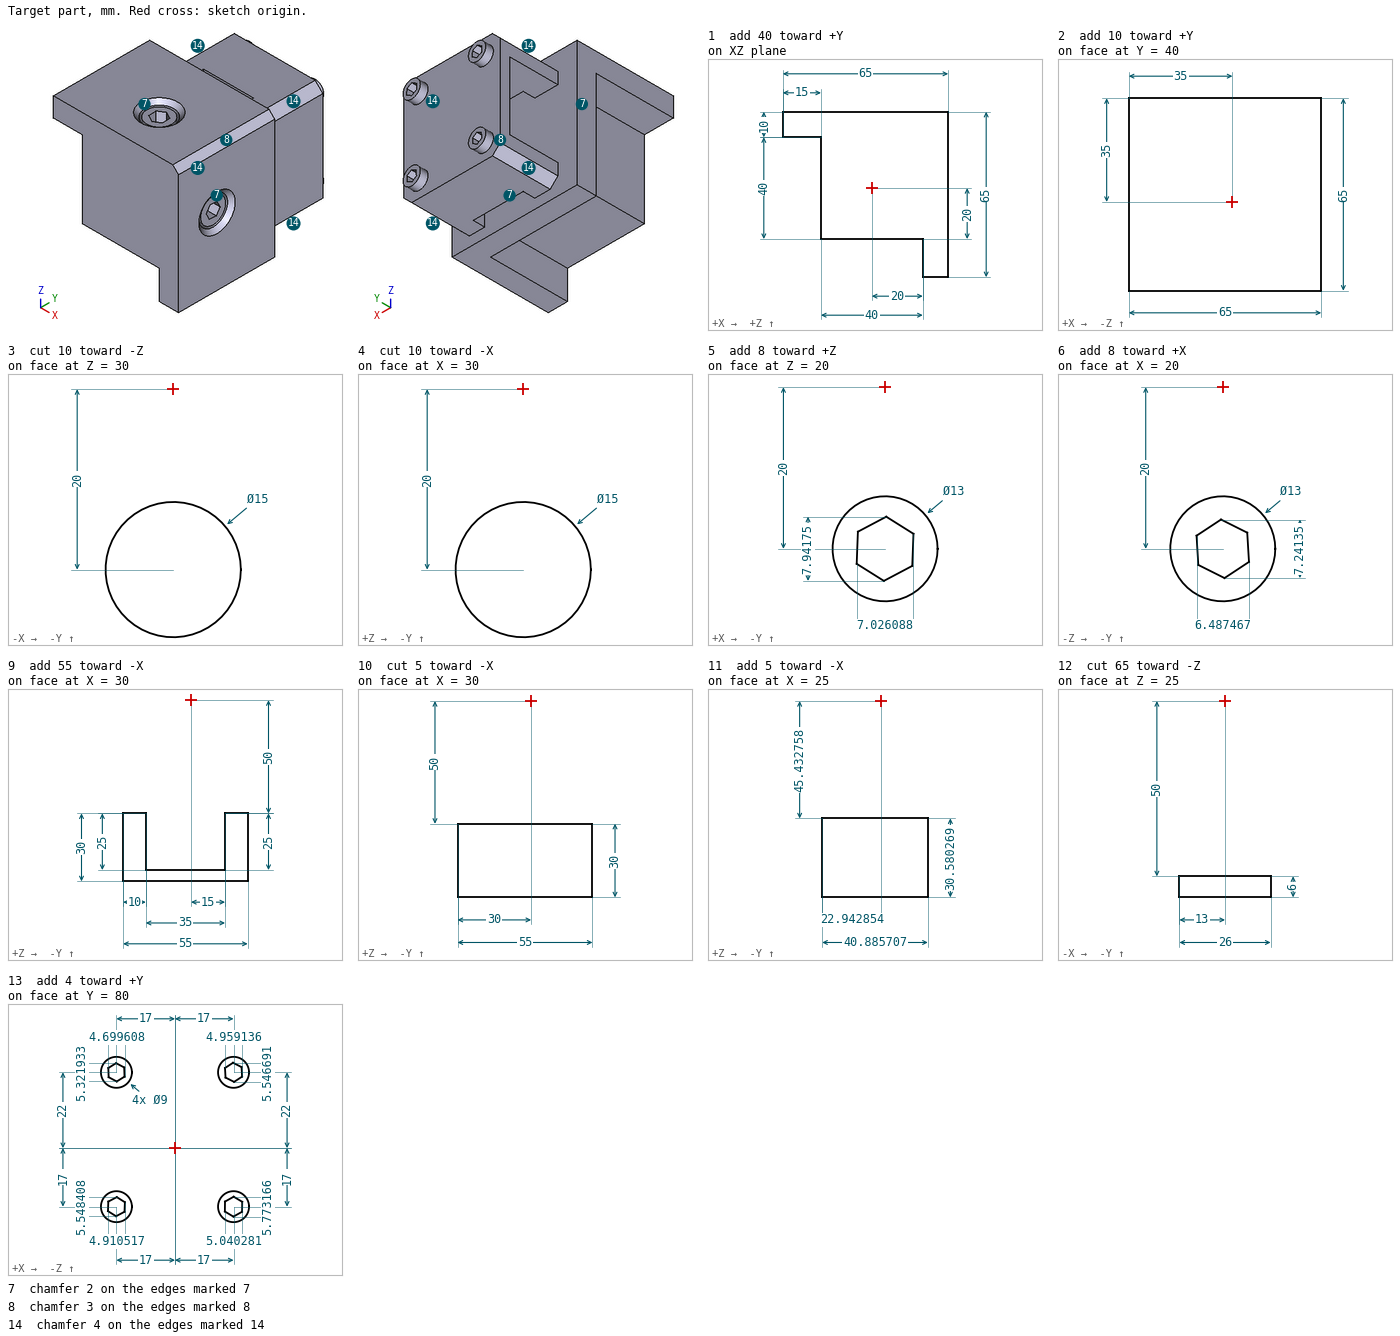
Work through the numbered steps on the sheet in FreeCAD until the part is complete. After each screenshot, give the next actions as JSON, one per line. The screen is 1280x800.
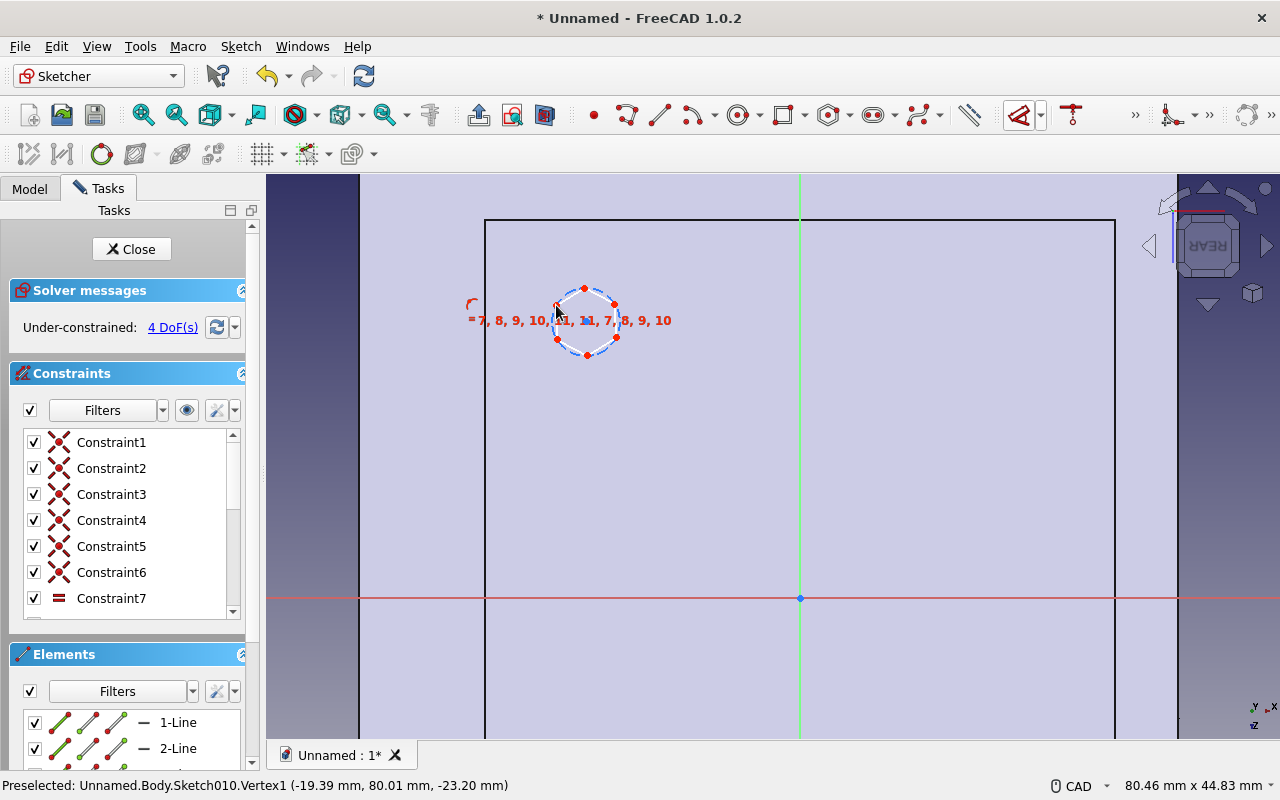
{"action": "left_click", "coordinate": [828, 116]}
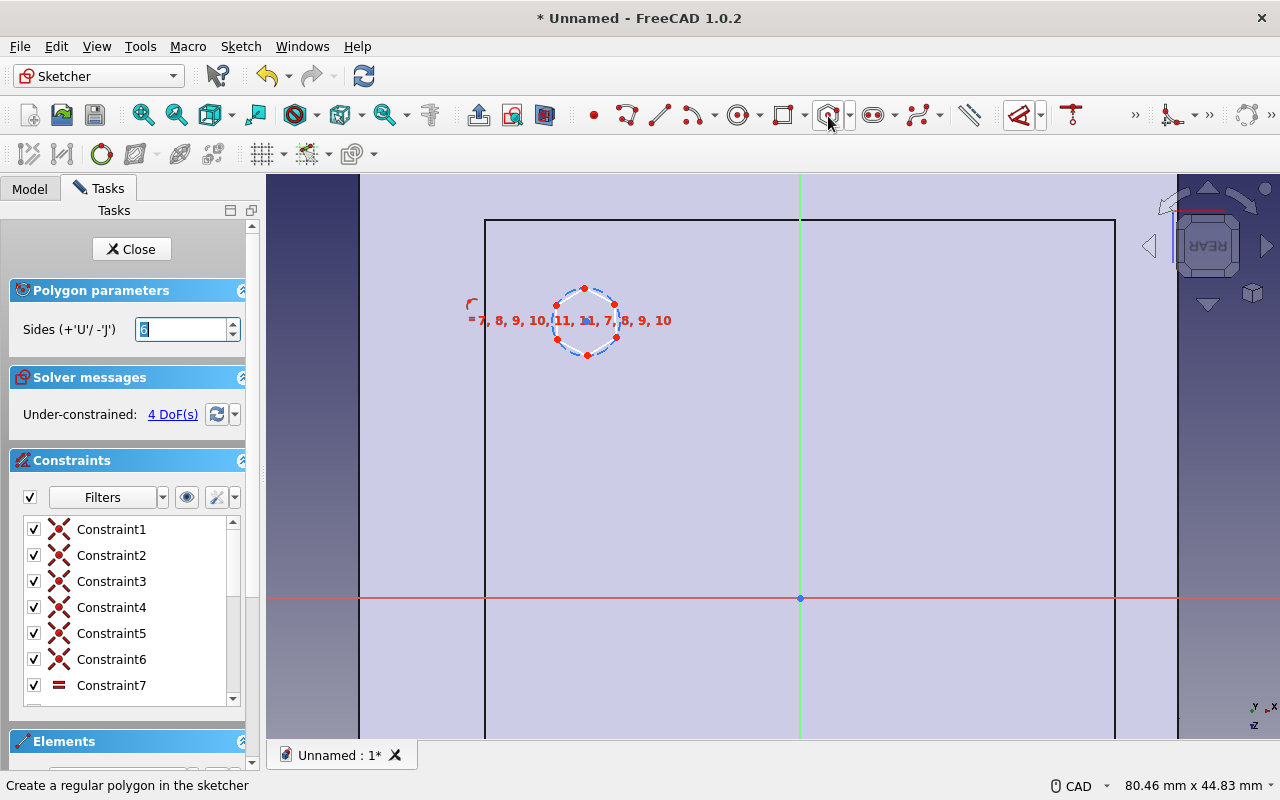
{"action": "left_click", "coordinate": [1015, 321]}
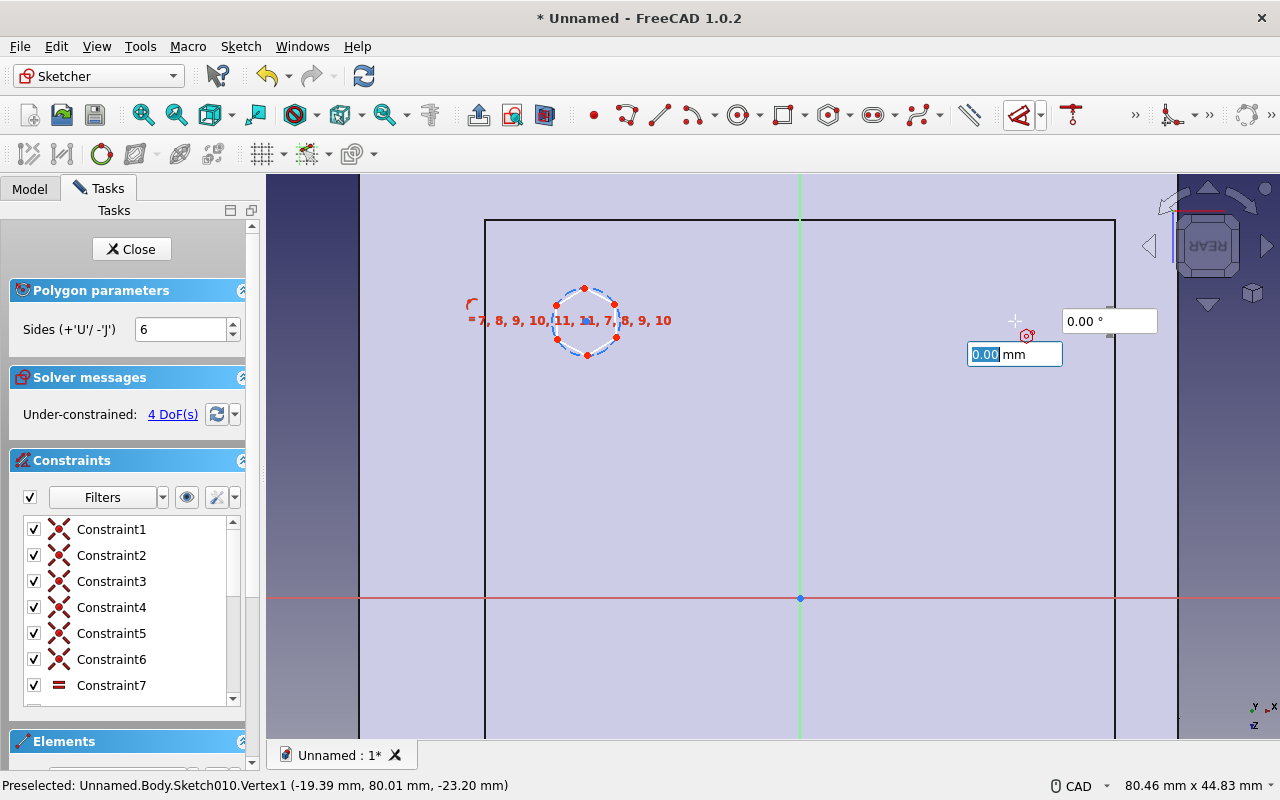
{"action": "left_click", "coordinate": [1046, 337]}
{"action": "right_click", "coordinate": [1046, 337]}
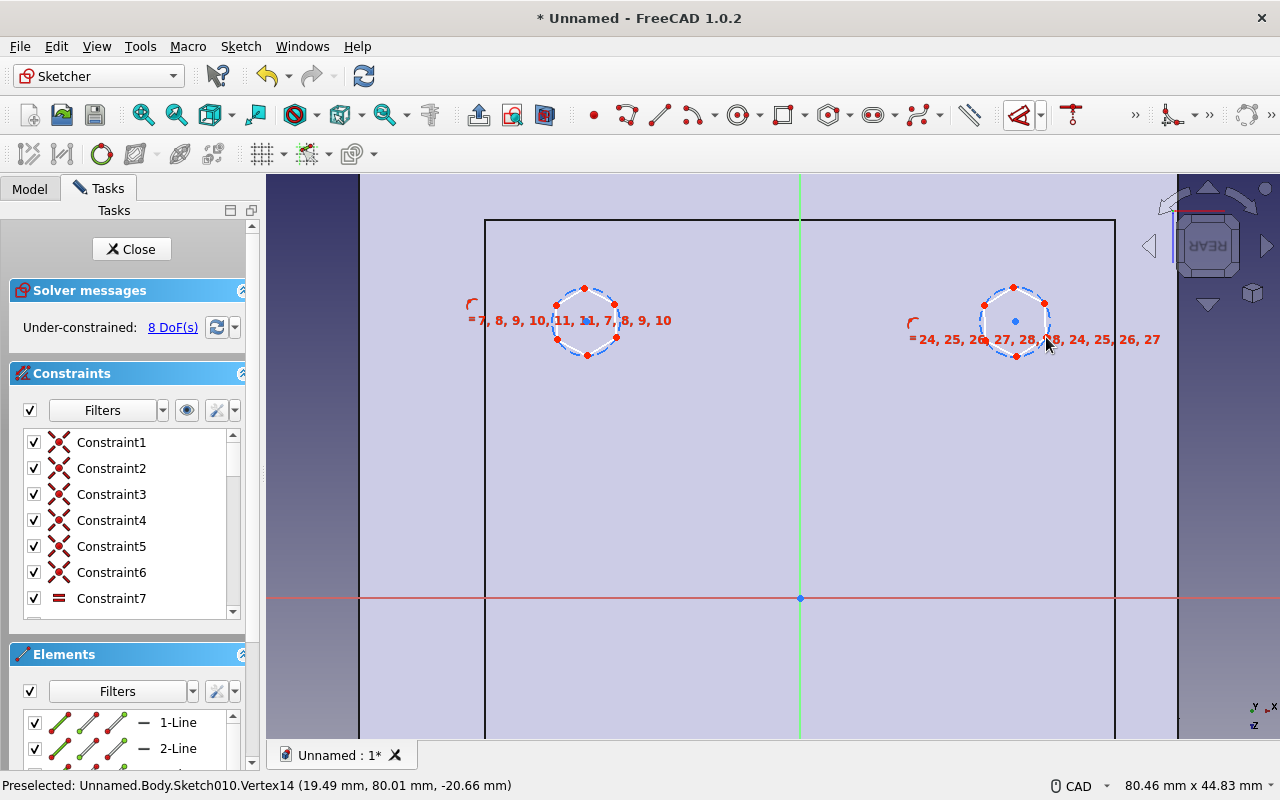
{"action": "left_click", "coordinate": [828, 116]}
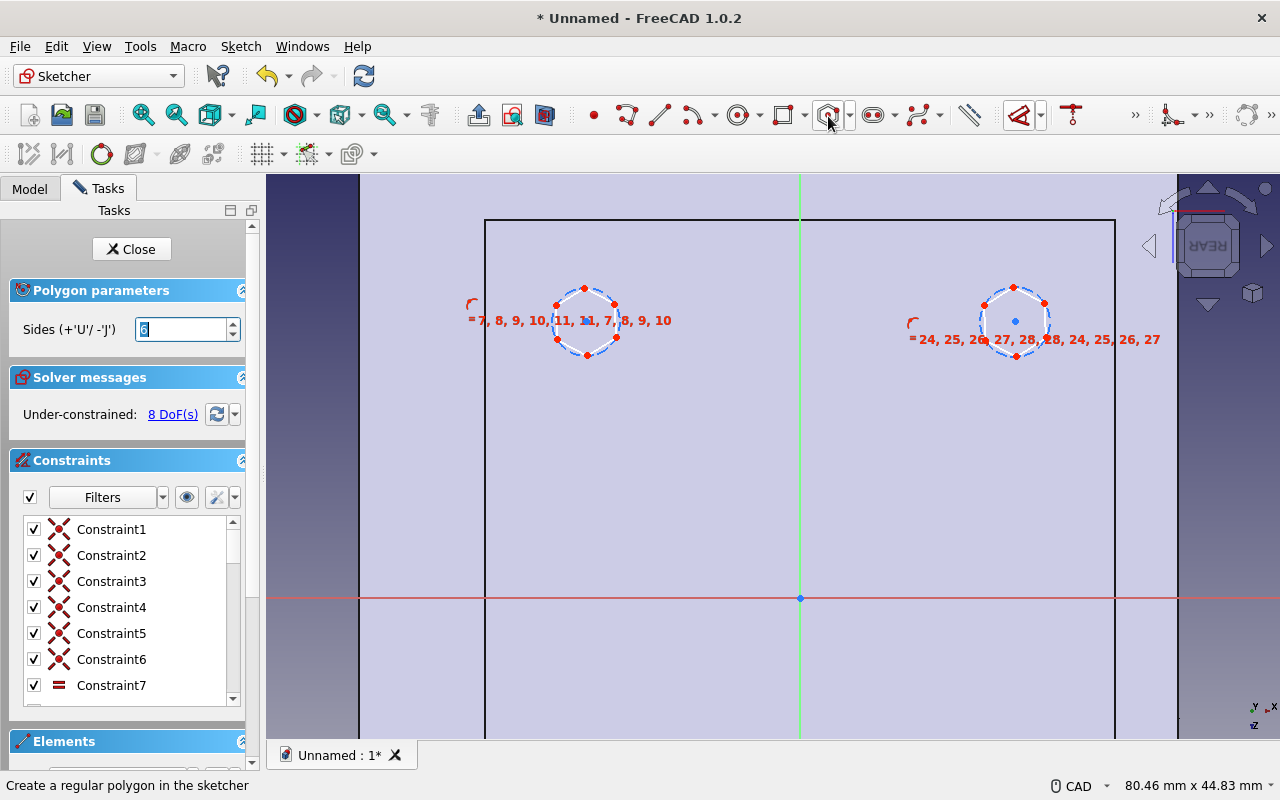
{"action": "scroll", "coordinate": [588, 322], "scroll_direction": "down", "scroll_amount": 3}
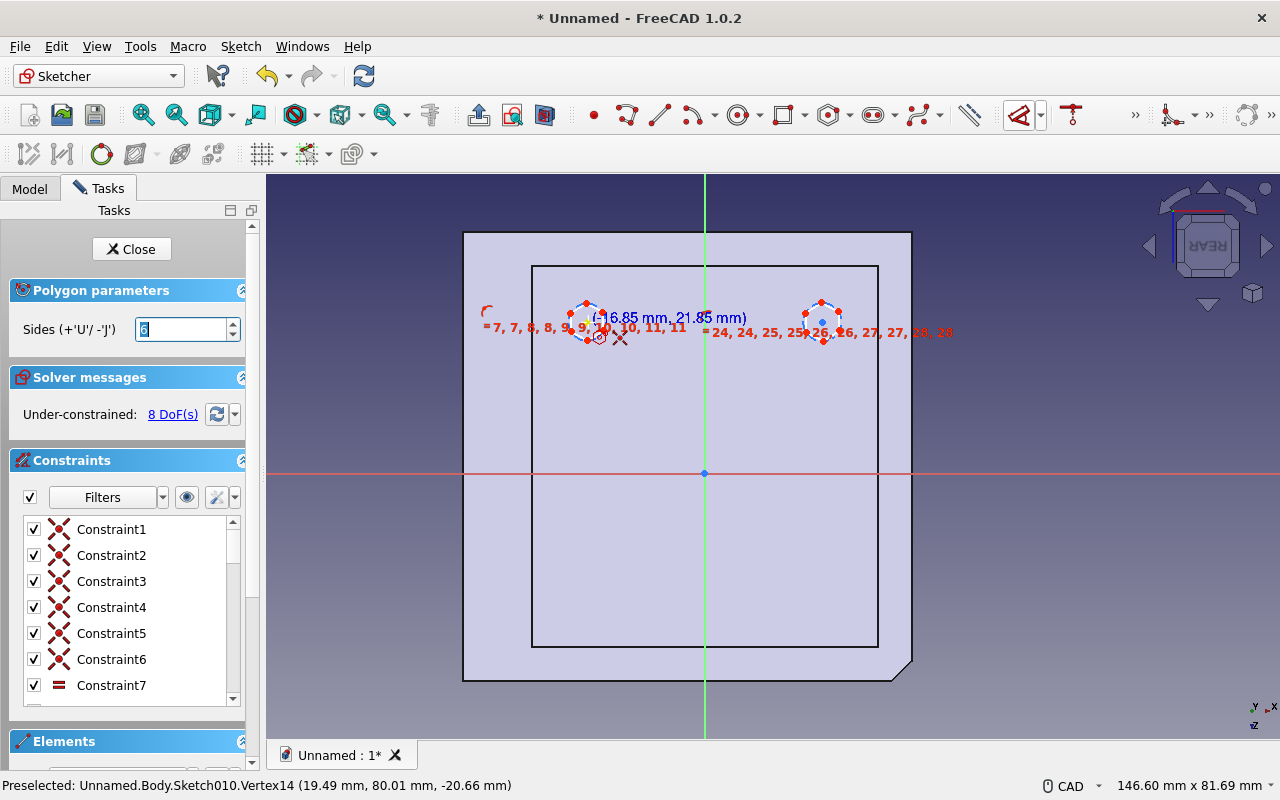
{"action": "scroll", "coordinate": [822, 591], "scroll_direction": "up", "scroll_amount": 3}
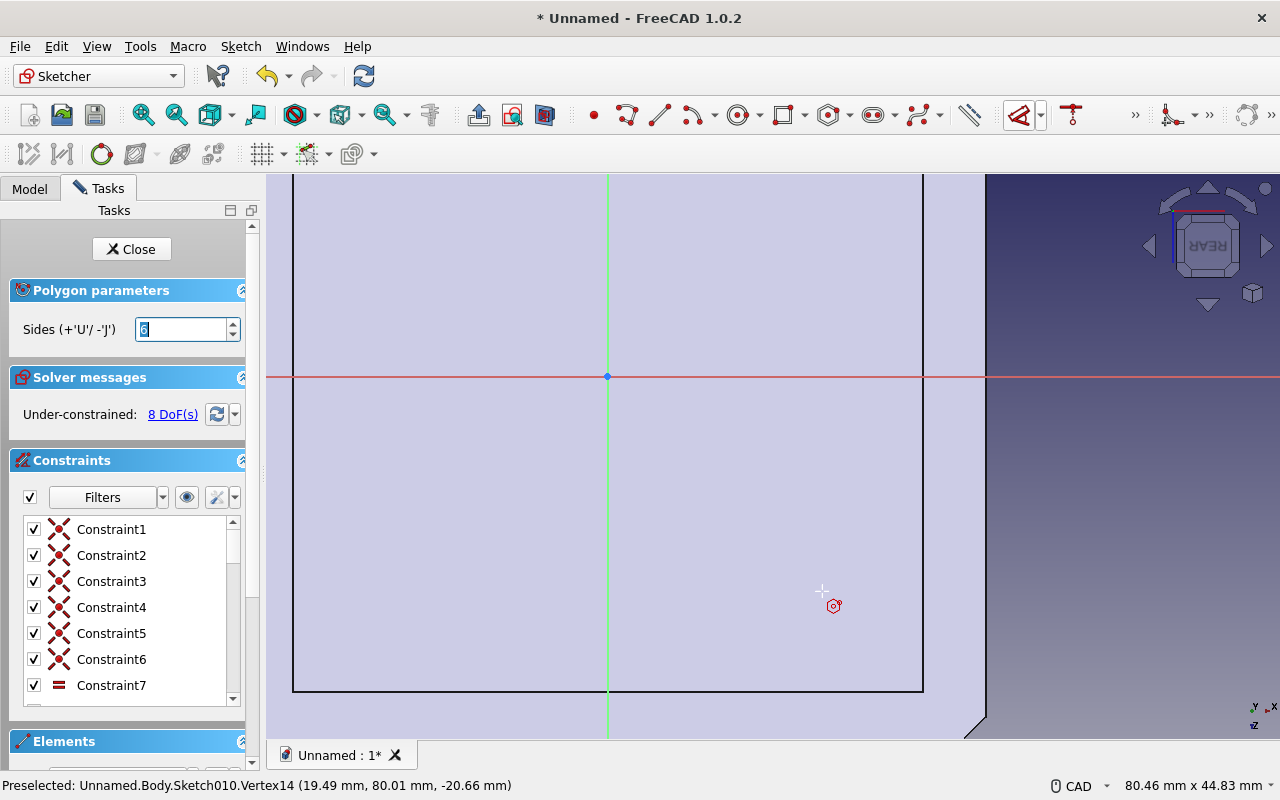
{"action": "left_click", "coordinate": [822, 591]}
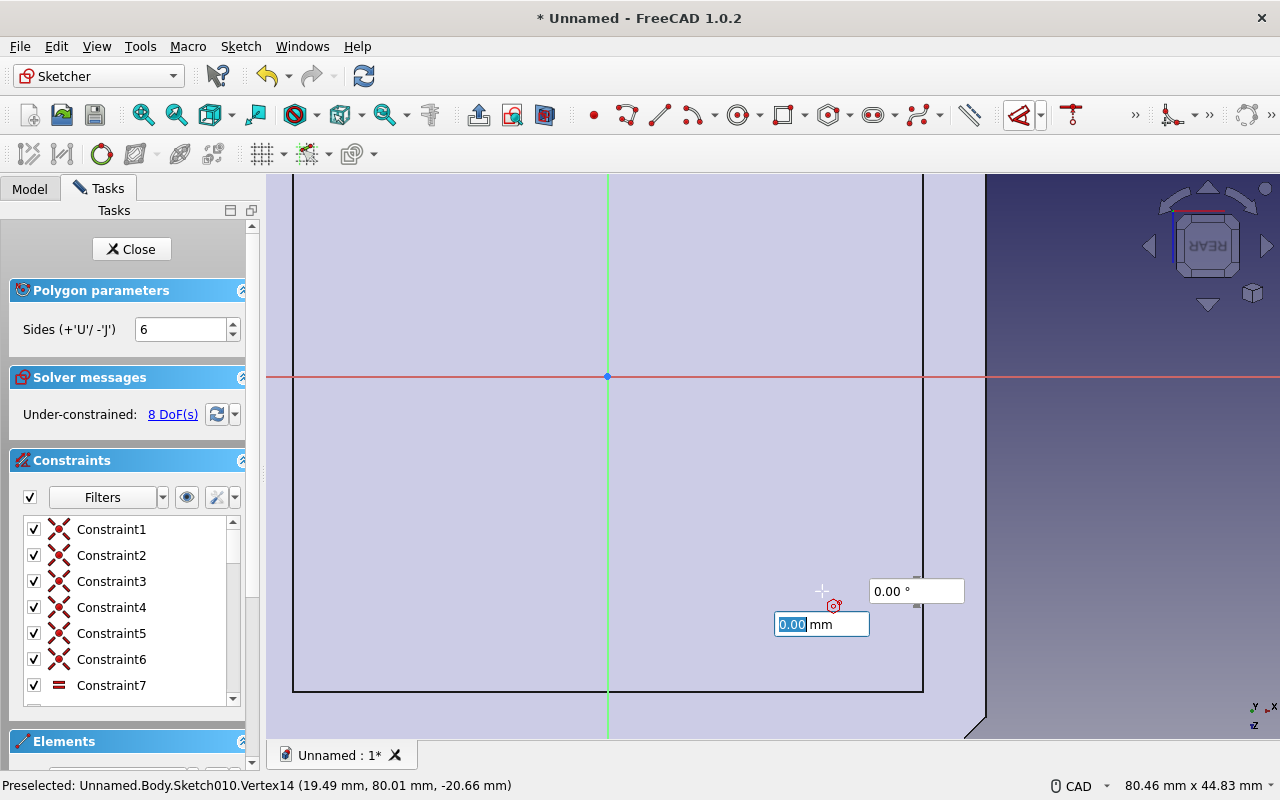
{"action": "left_click", "coordinate": [853, 610]}
{"action": "right_click", "coordinate": [853, 610]}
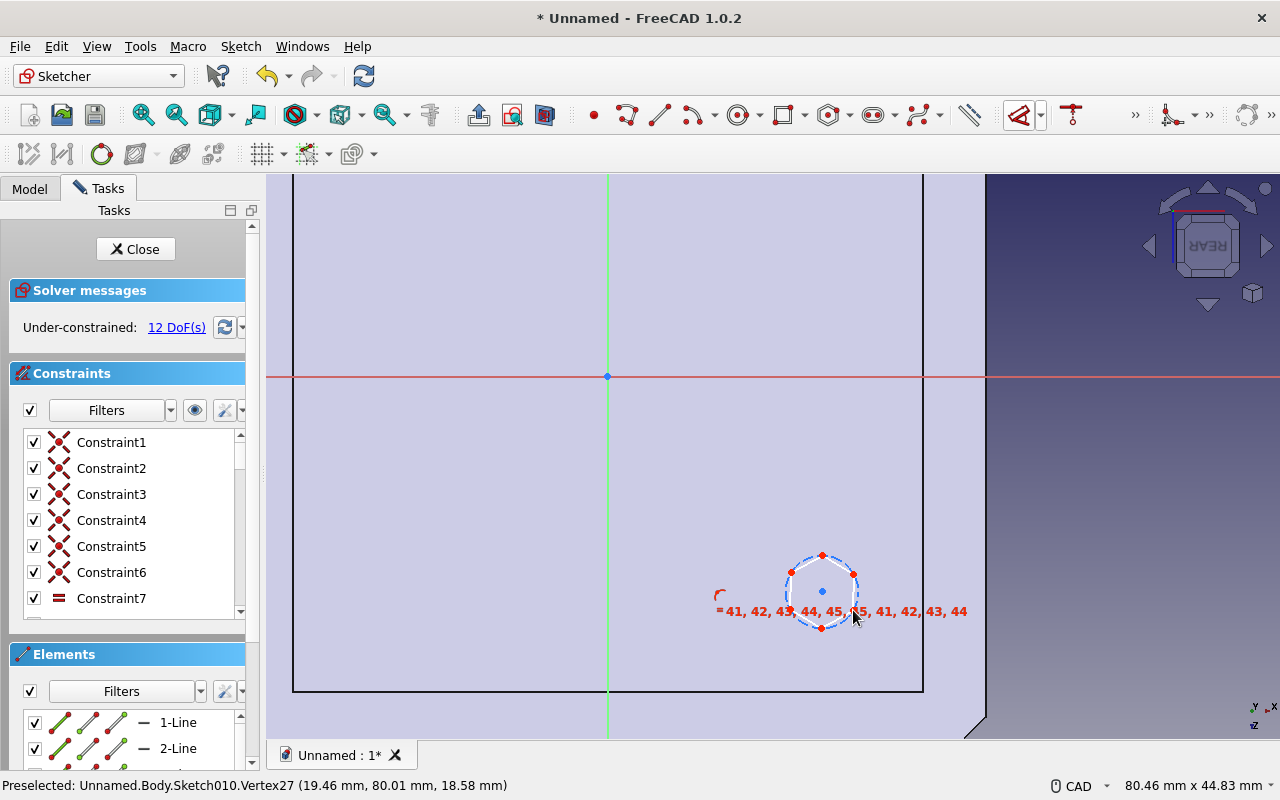
{"action": "left_click", "coordinate": [828, 116]}